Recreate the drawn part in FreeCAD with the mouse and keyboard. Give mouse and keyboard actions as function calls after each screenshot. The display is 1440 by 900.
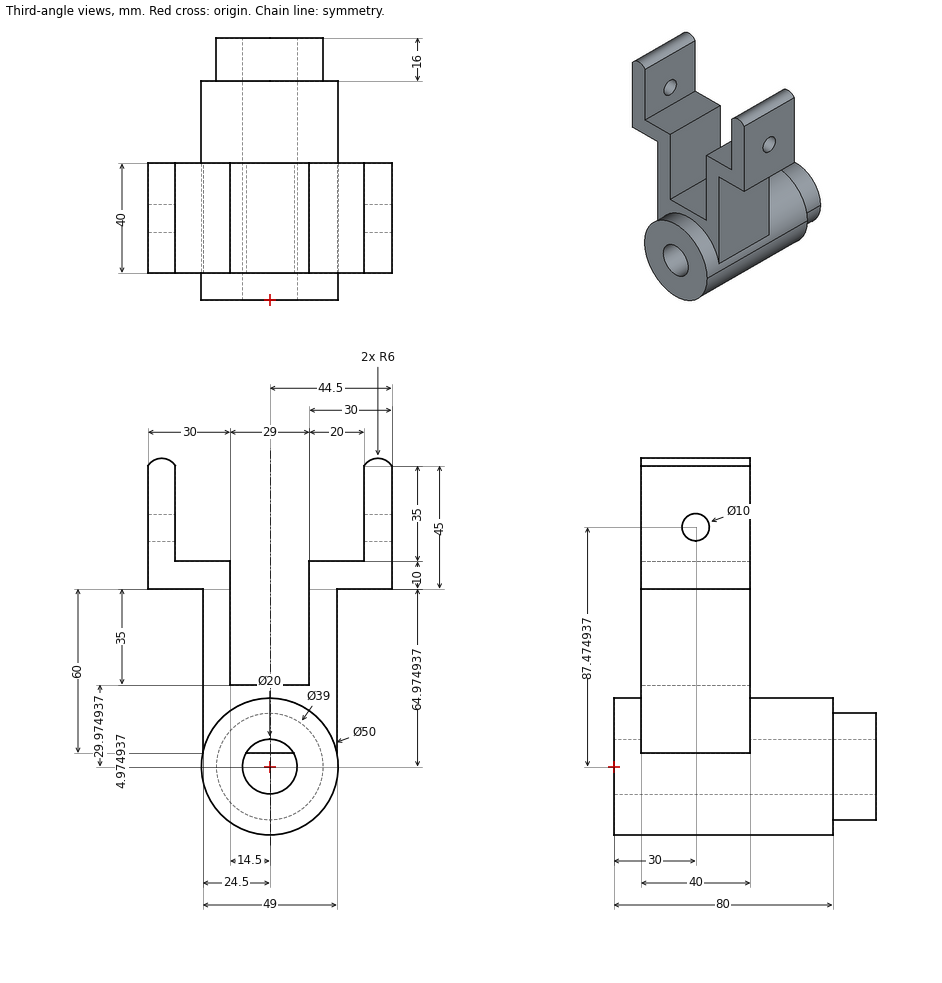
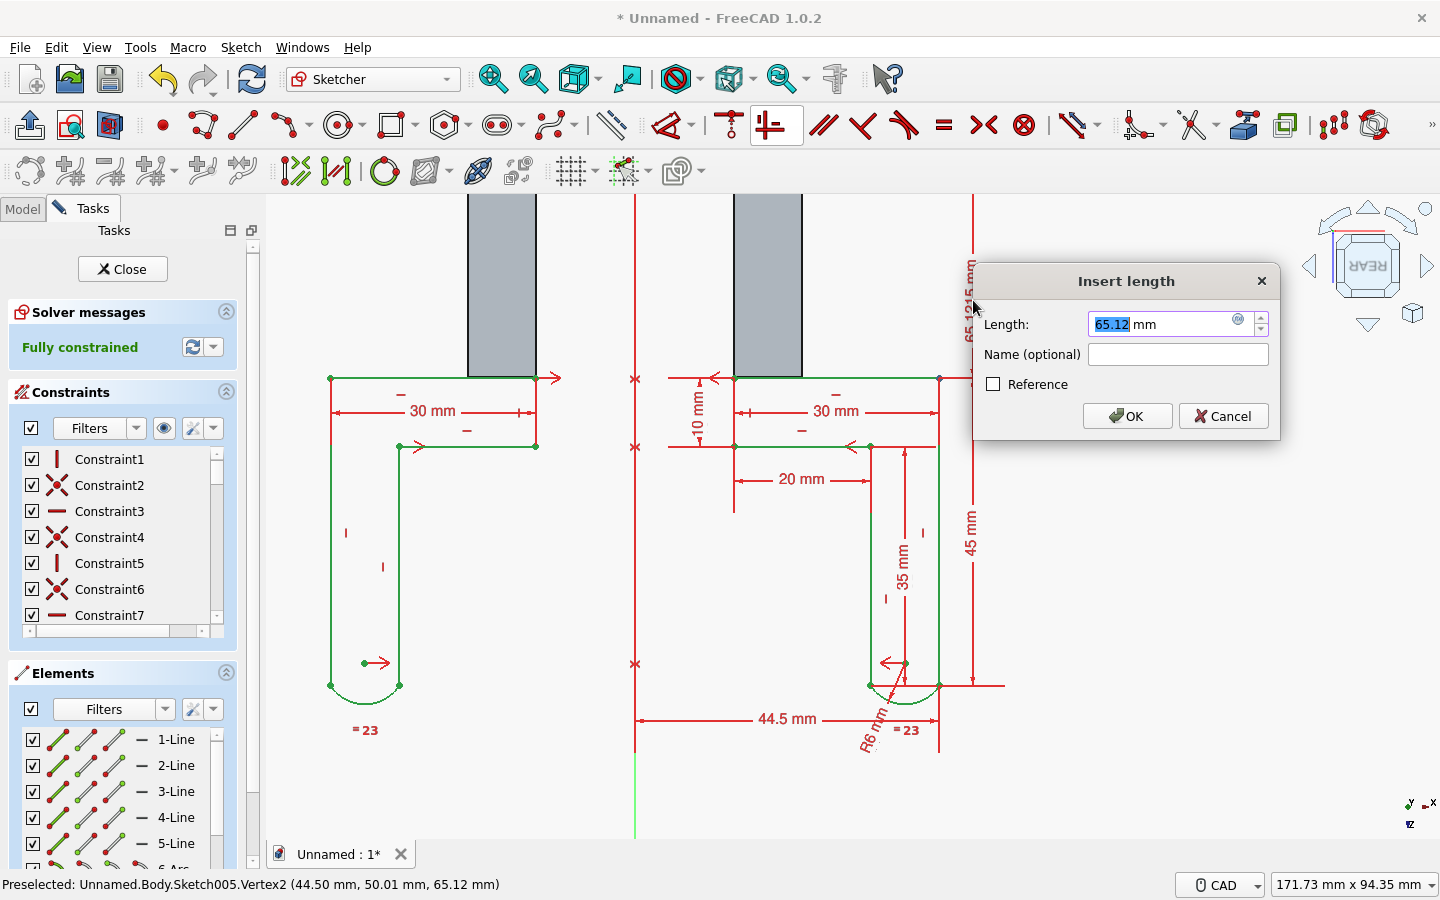
text(64.974937)
key(Return)
key(Escape)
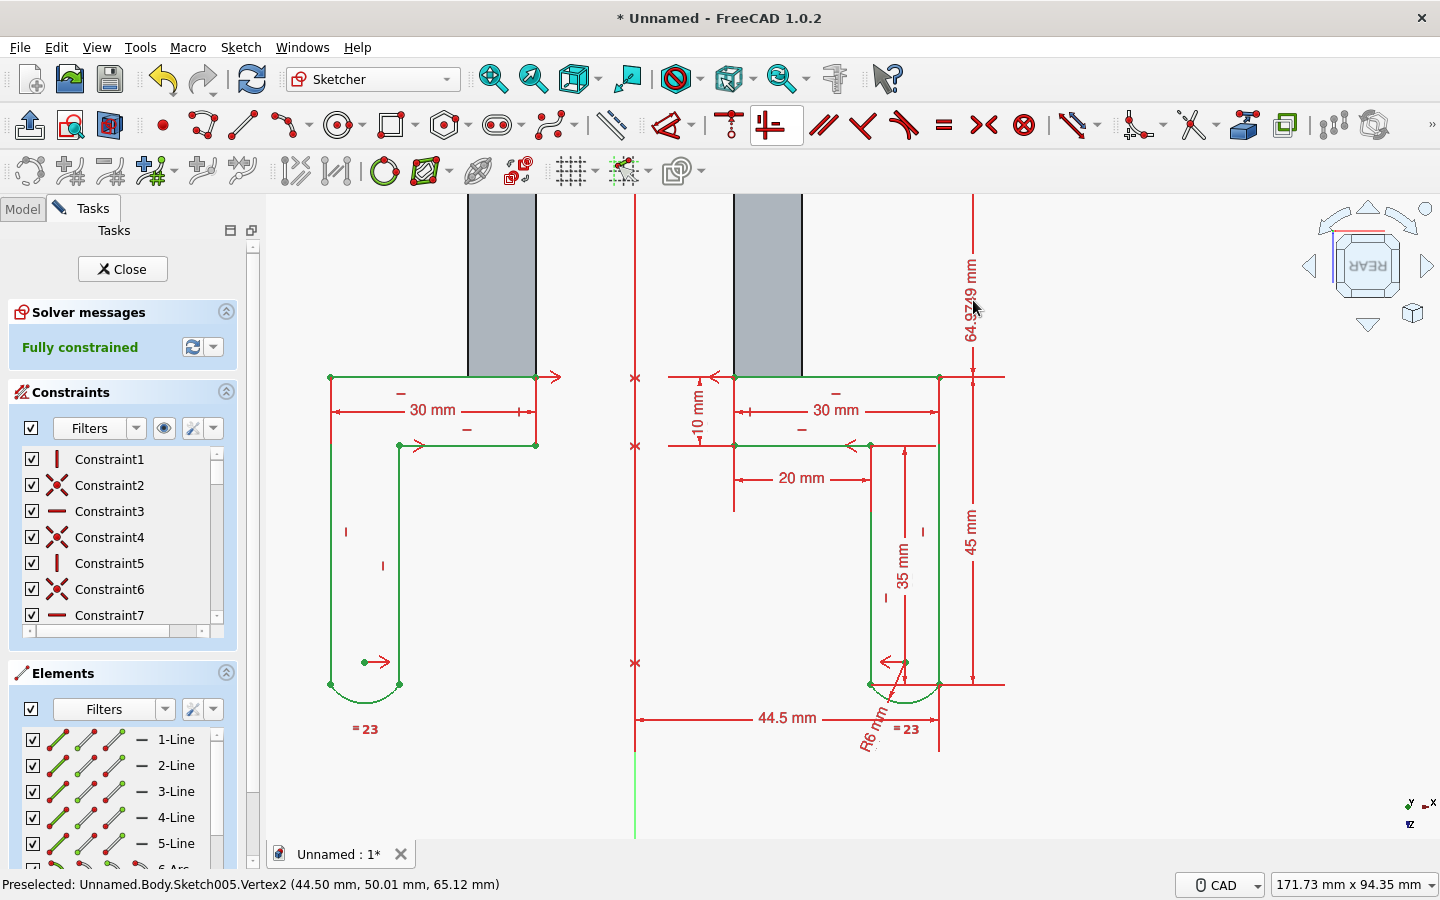
click(123, 269)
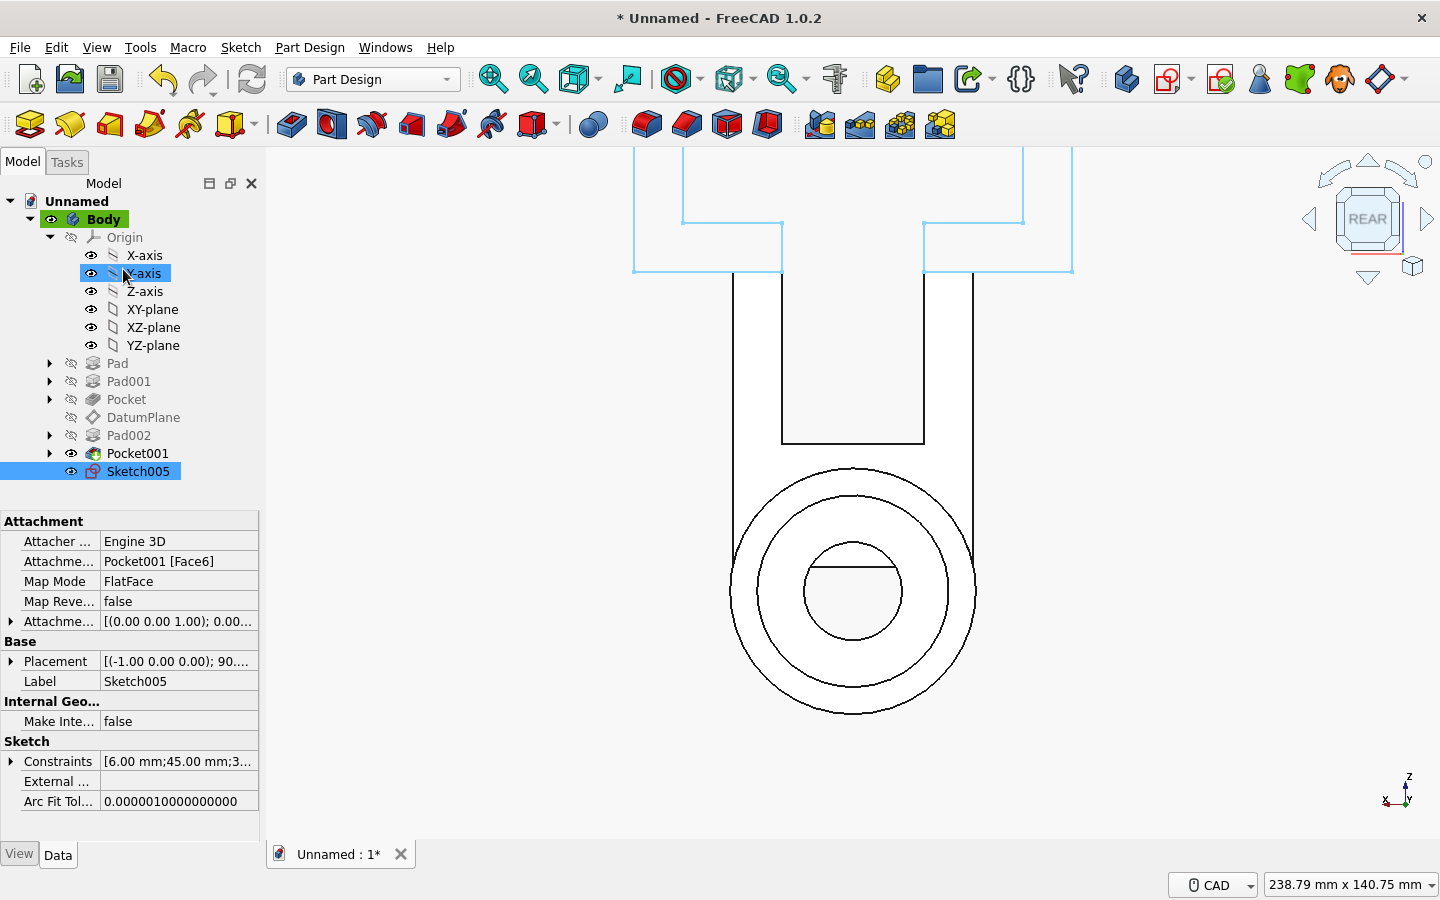
click(30, 124)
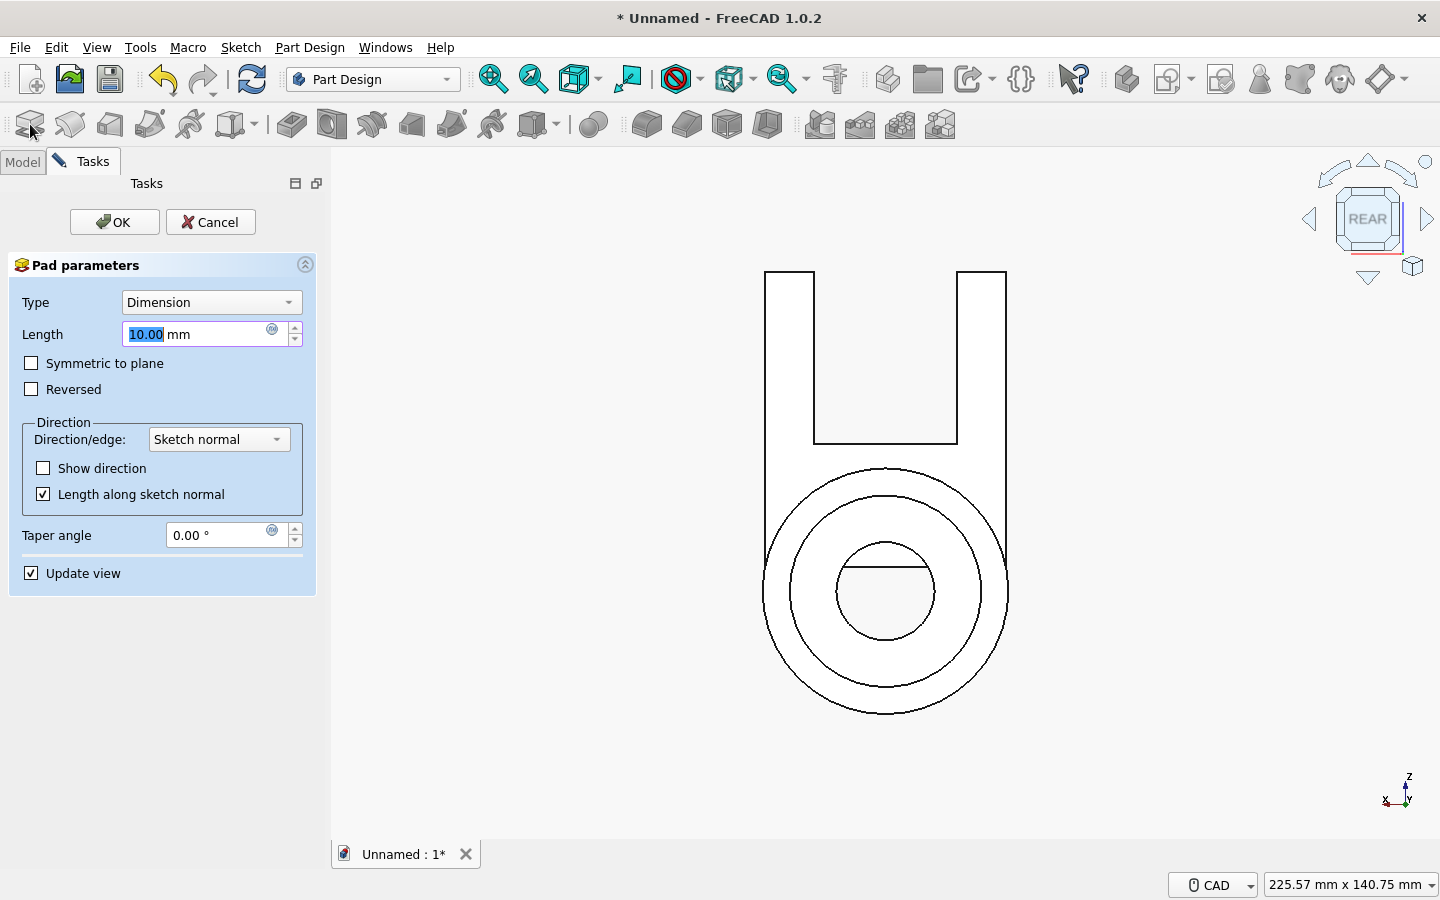
text(40)
key(Tab)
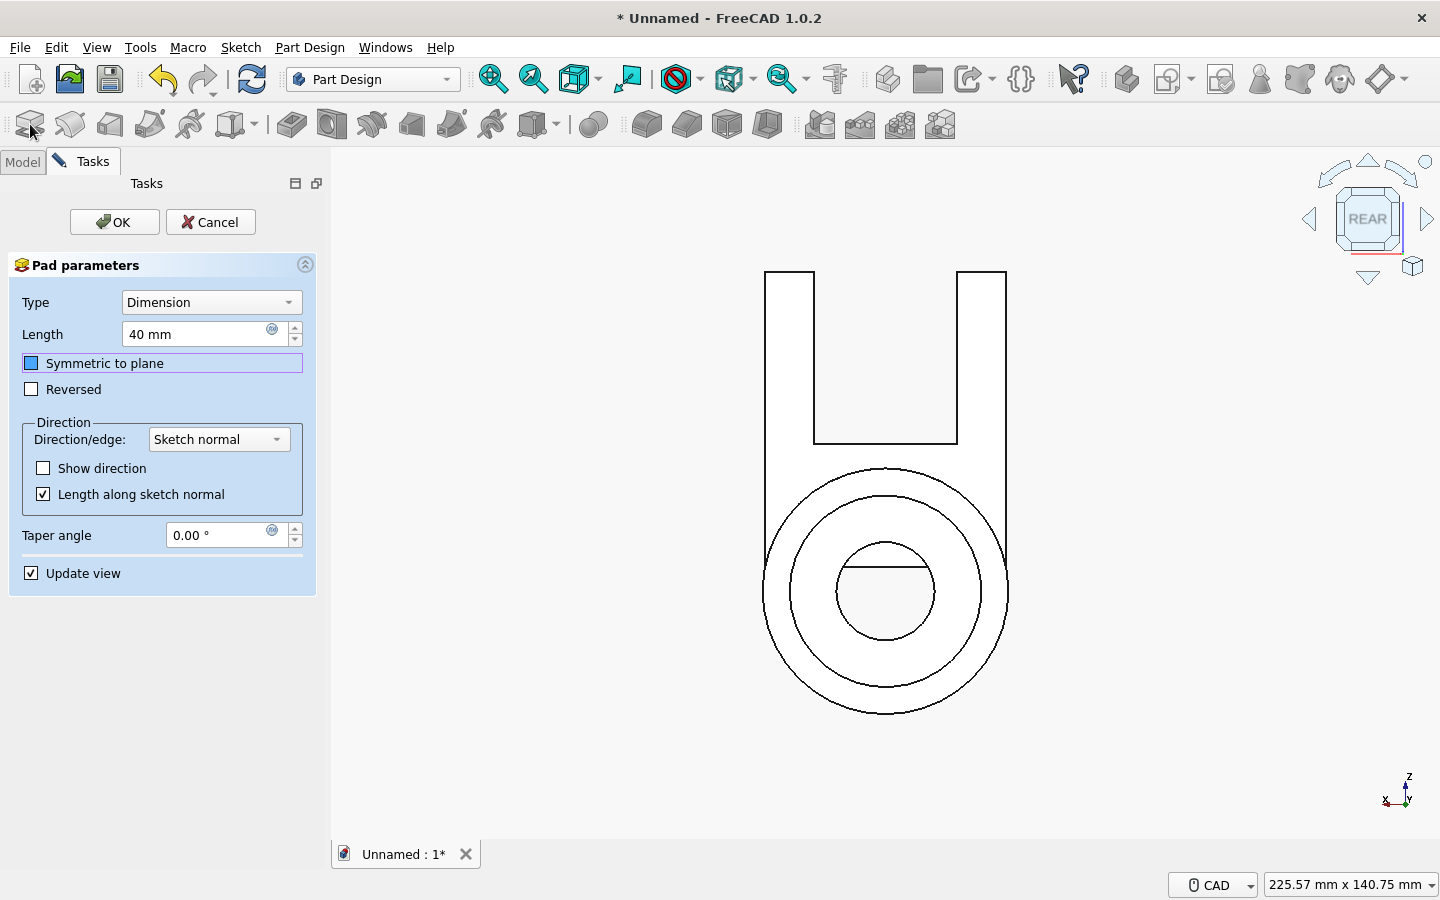
click(30, 389)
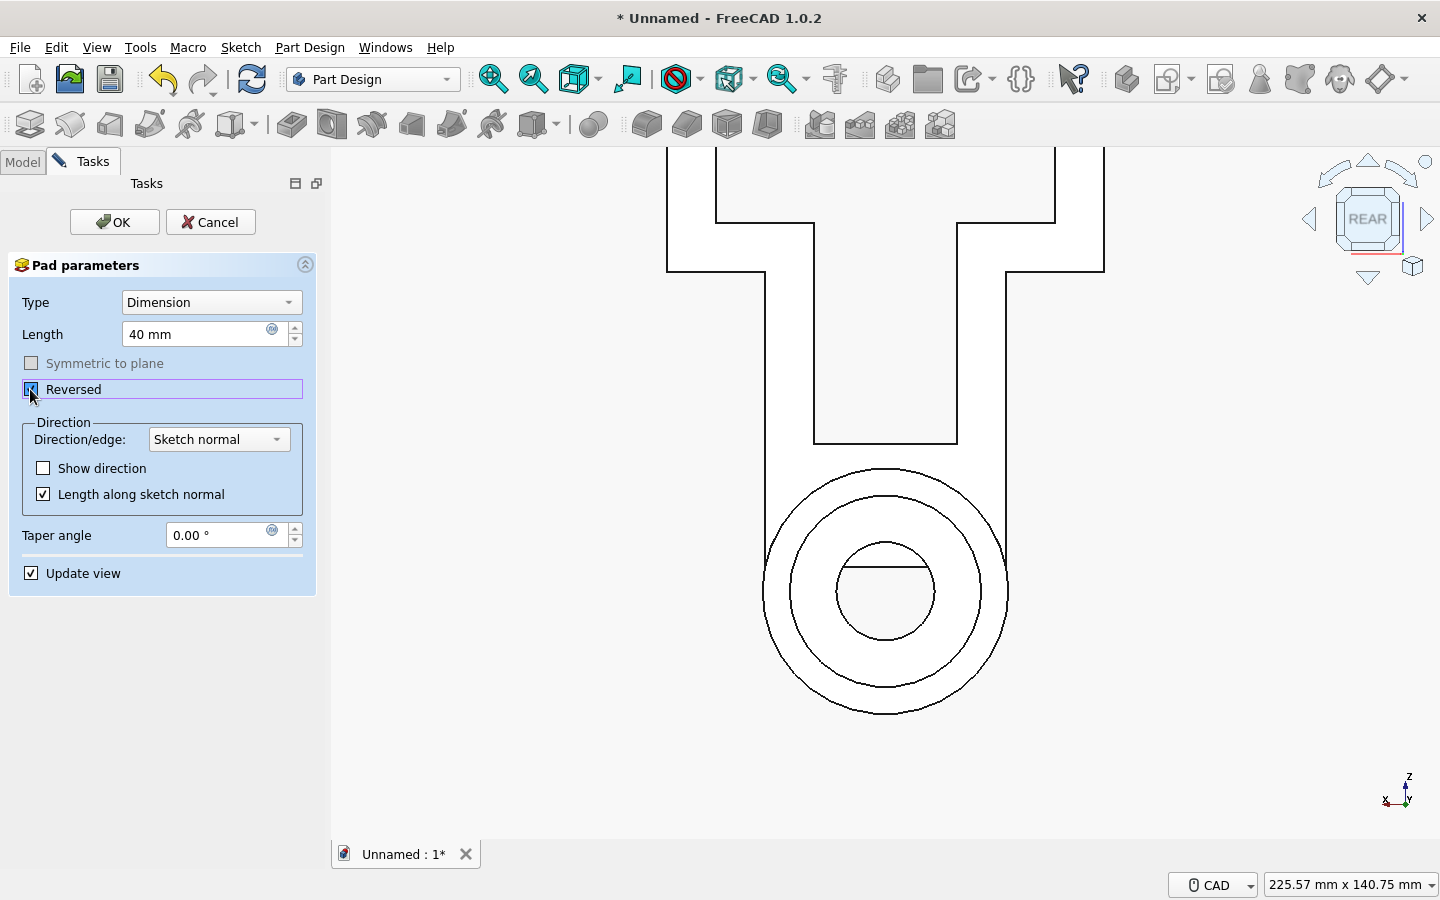
click(115, 222)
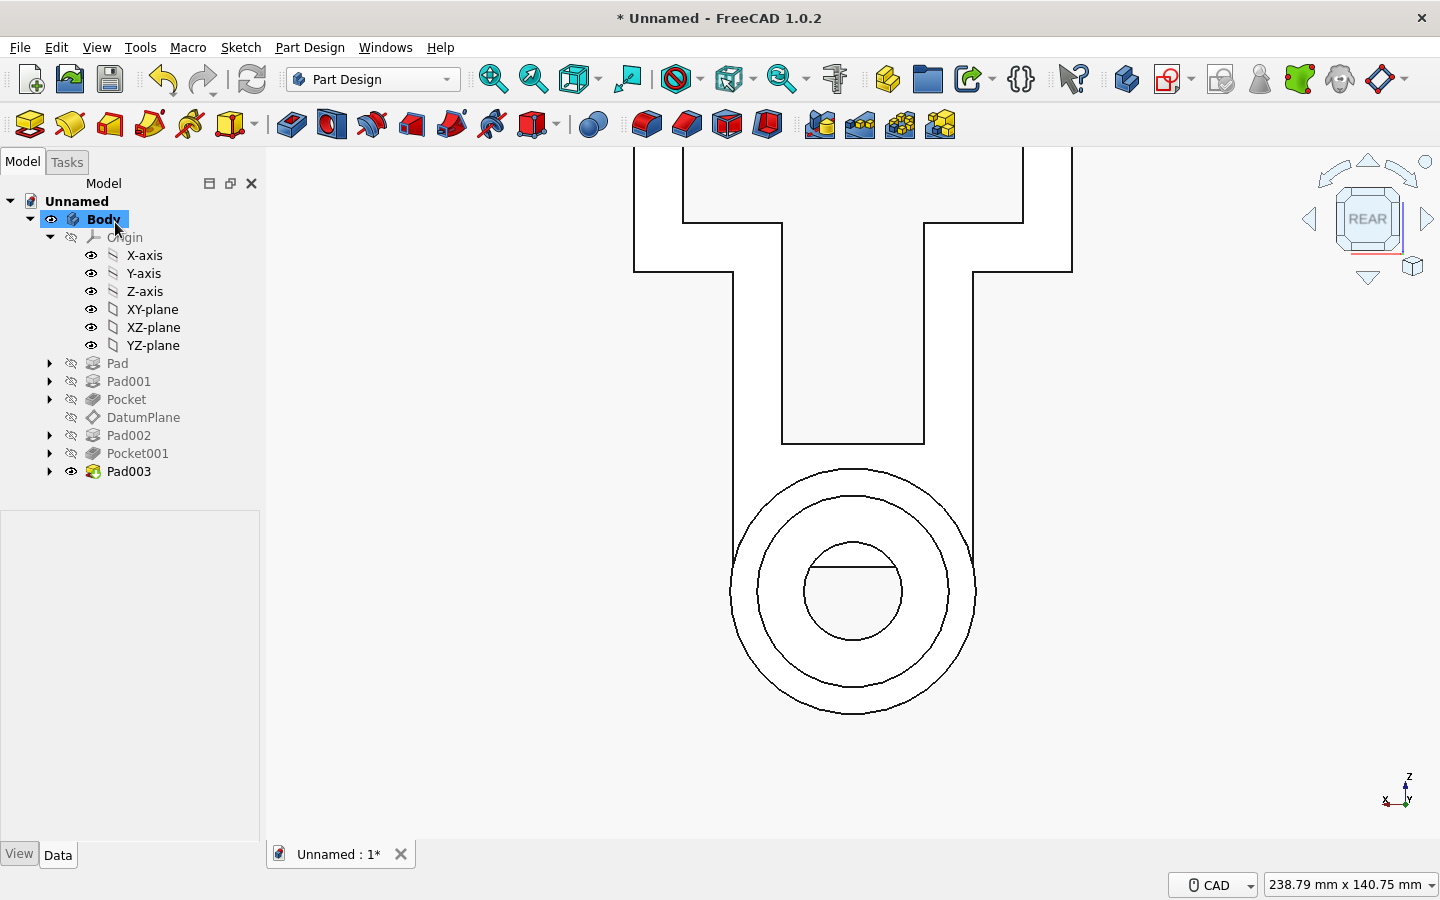
click(494, 80)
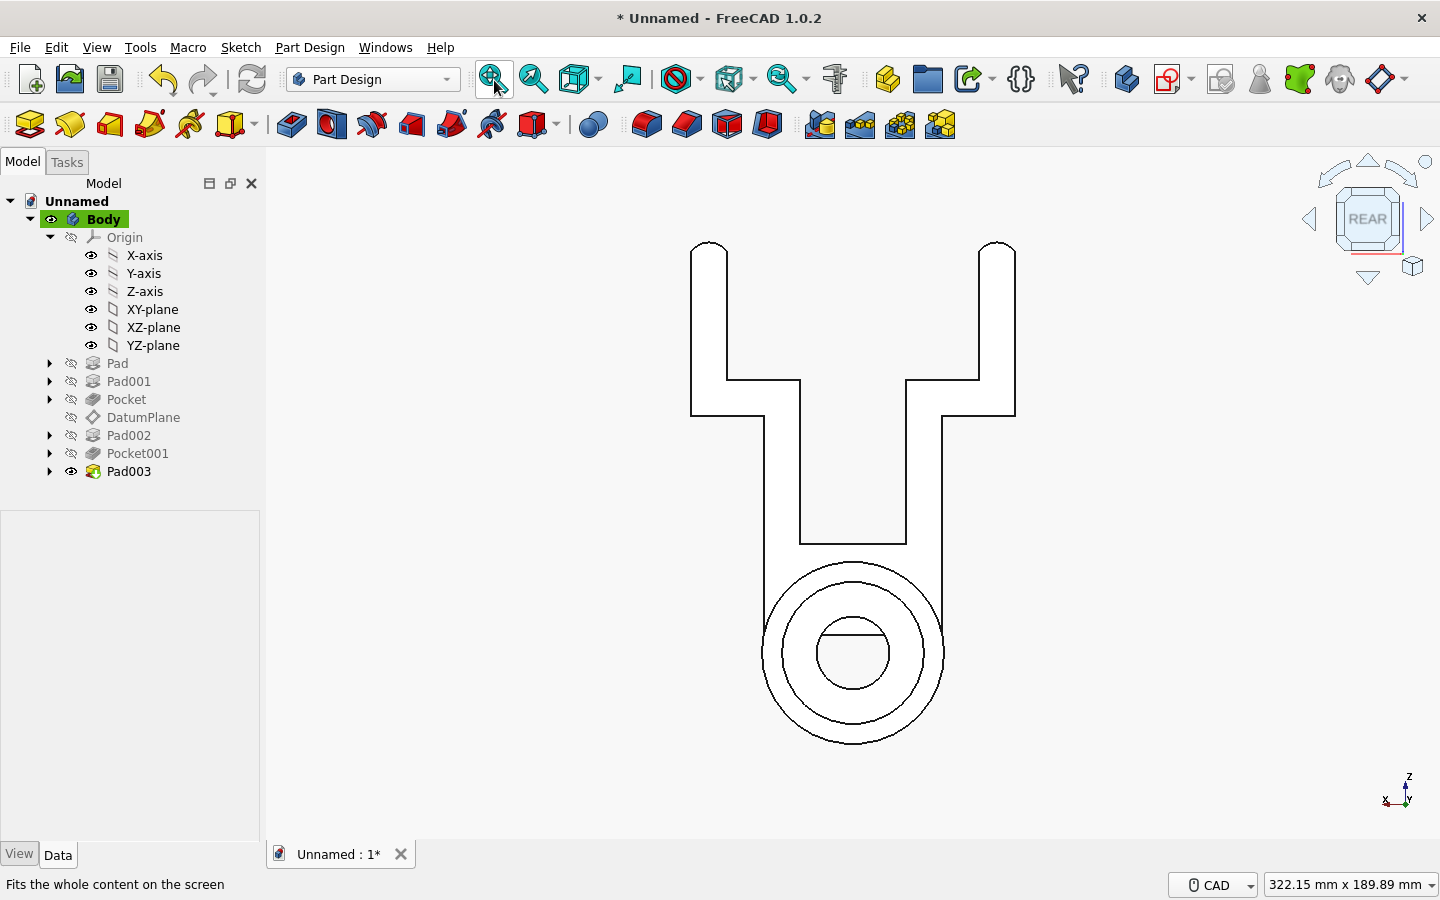
key(0)